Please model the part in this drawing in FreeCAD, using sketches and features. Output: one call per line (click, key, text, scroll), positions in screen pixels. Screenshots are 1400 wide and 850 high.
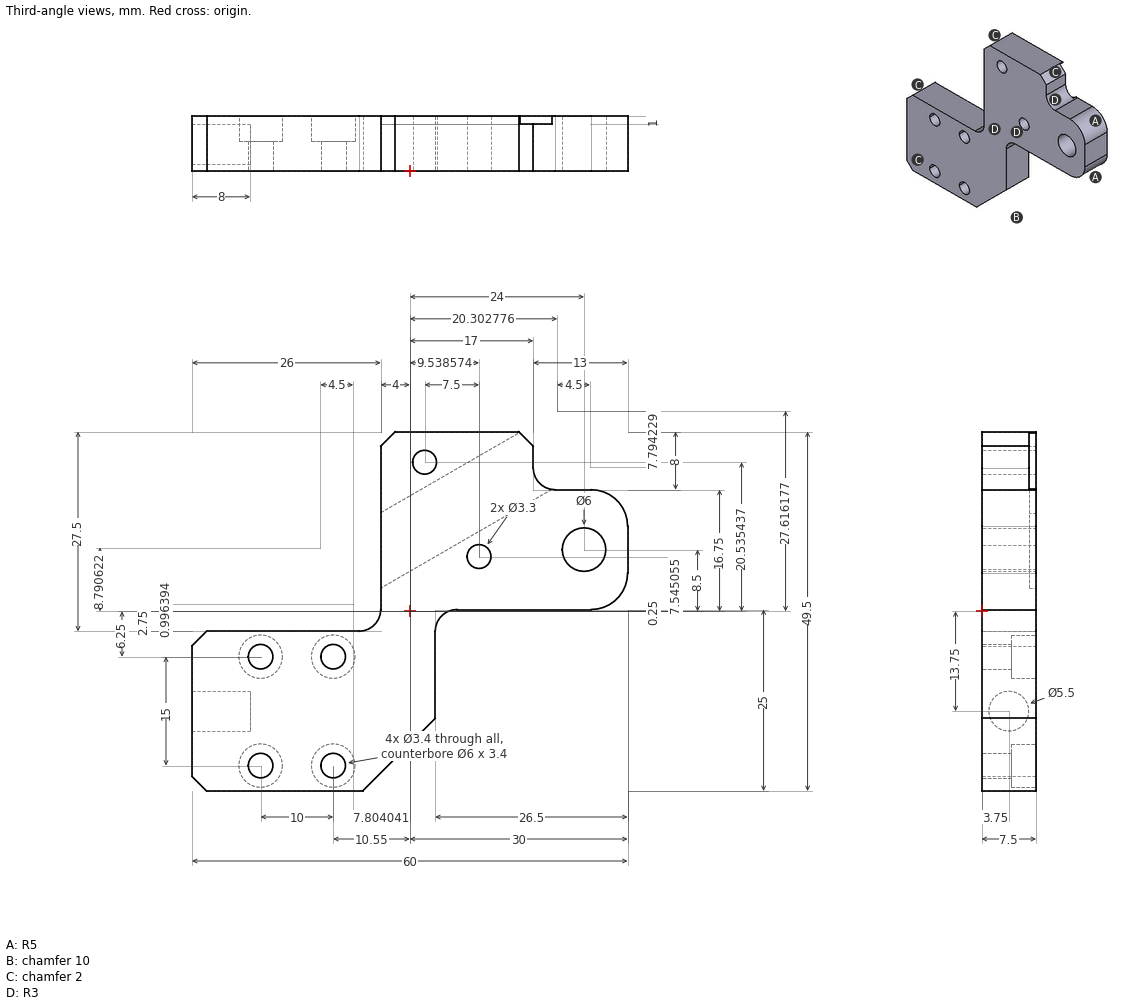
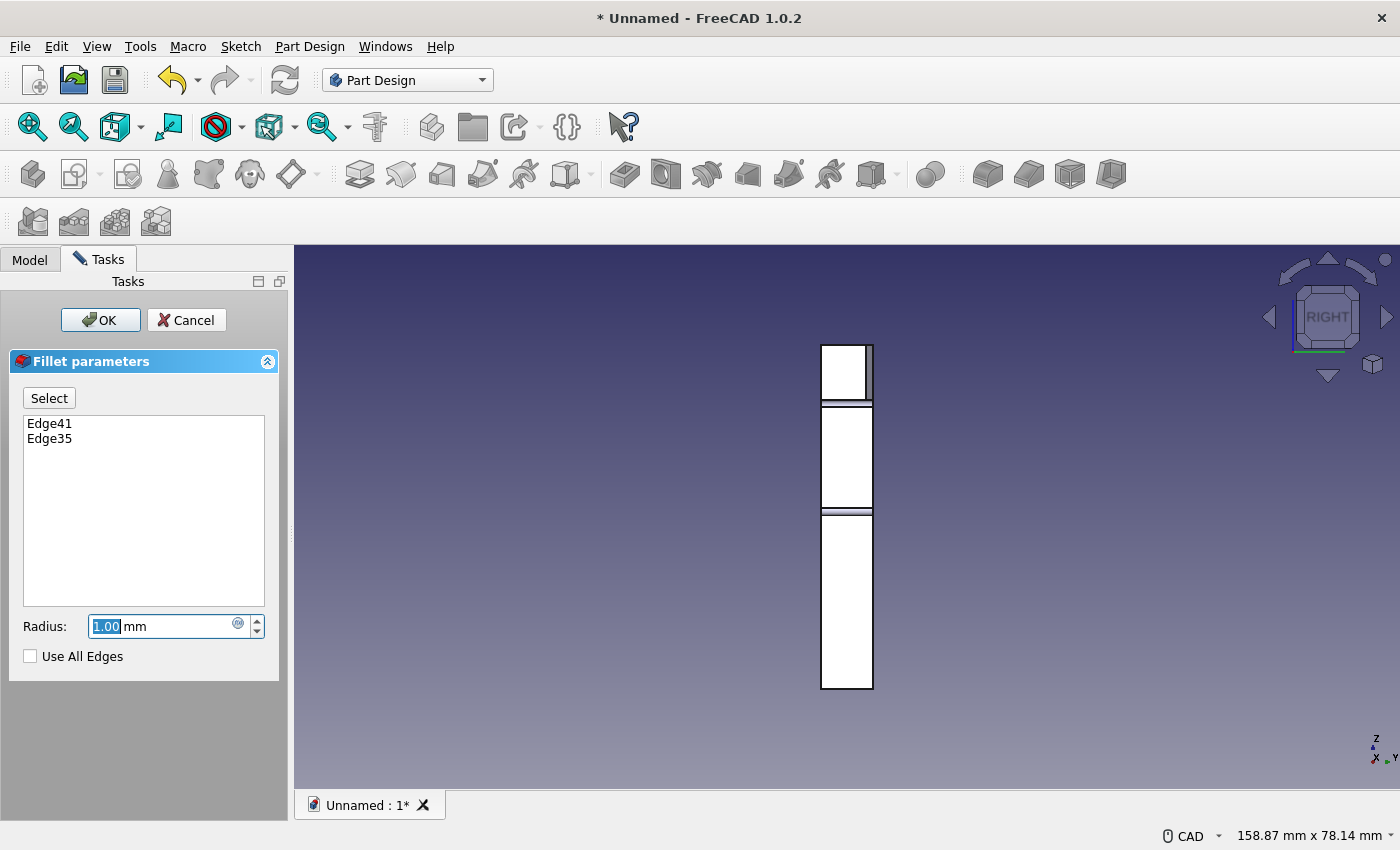
text(5)
key(Tab)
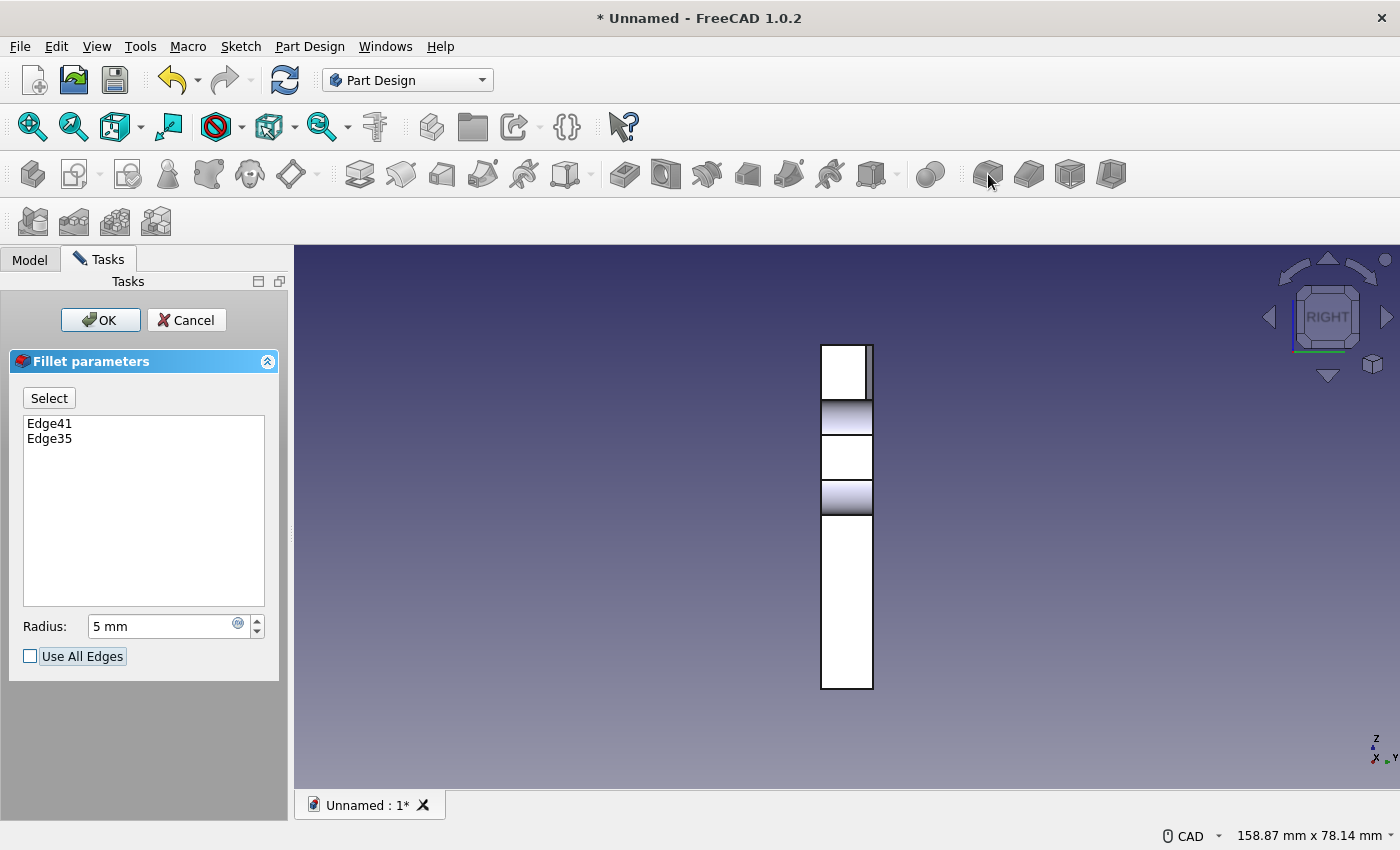
click(101, 320)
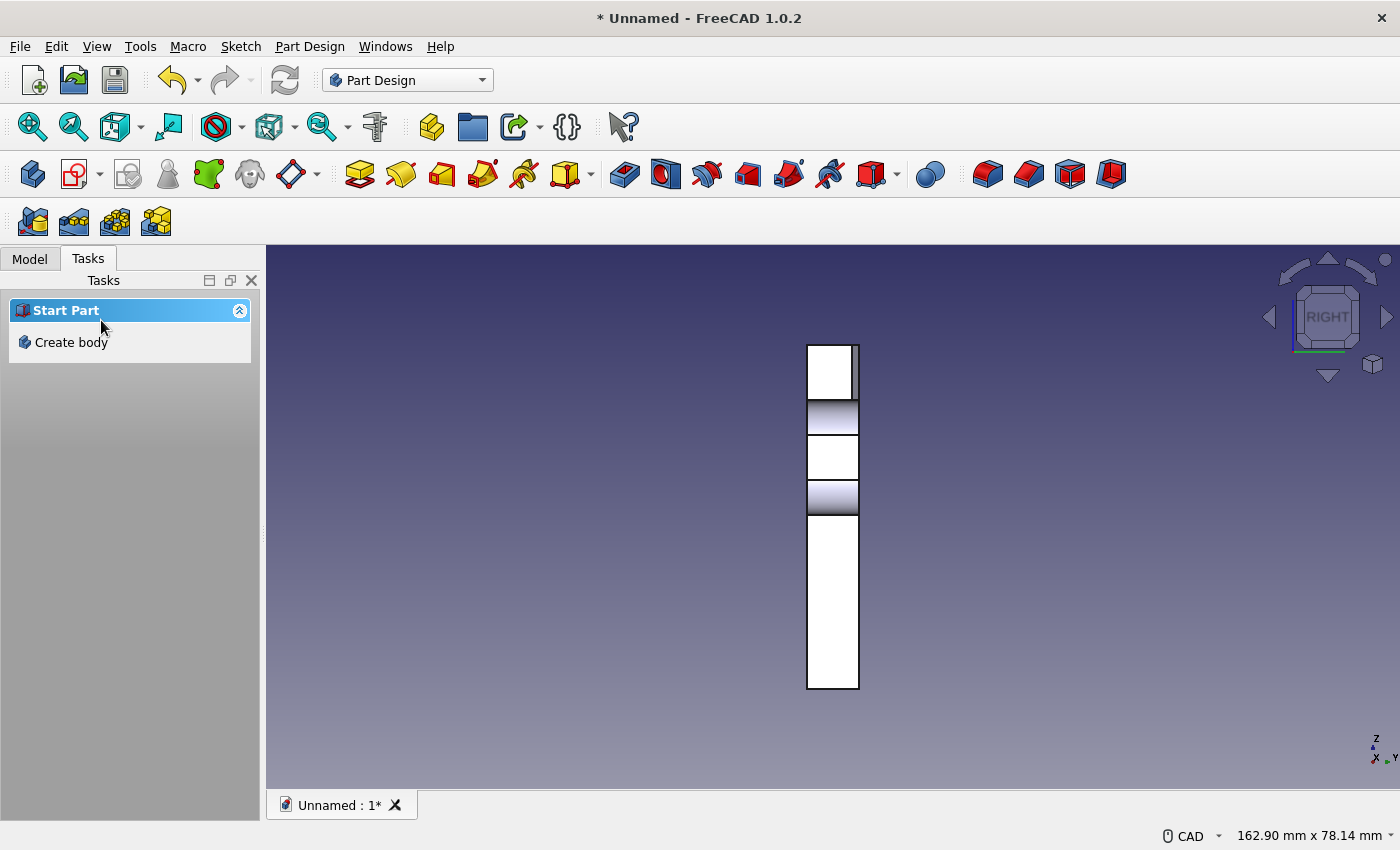
click(833, 688)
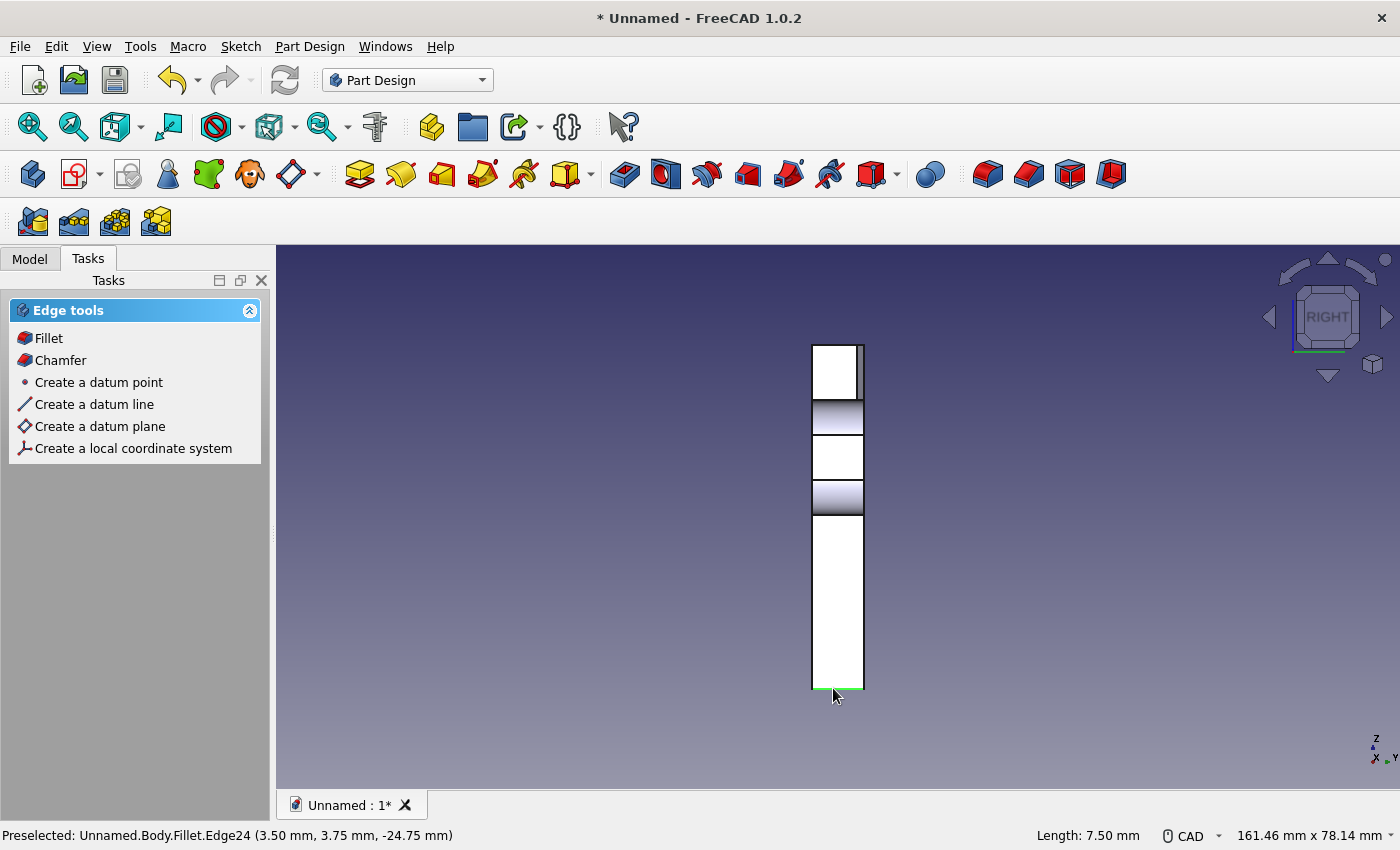
click(1029, 174)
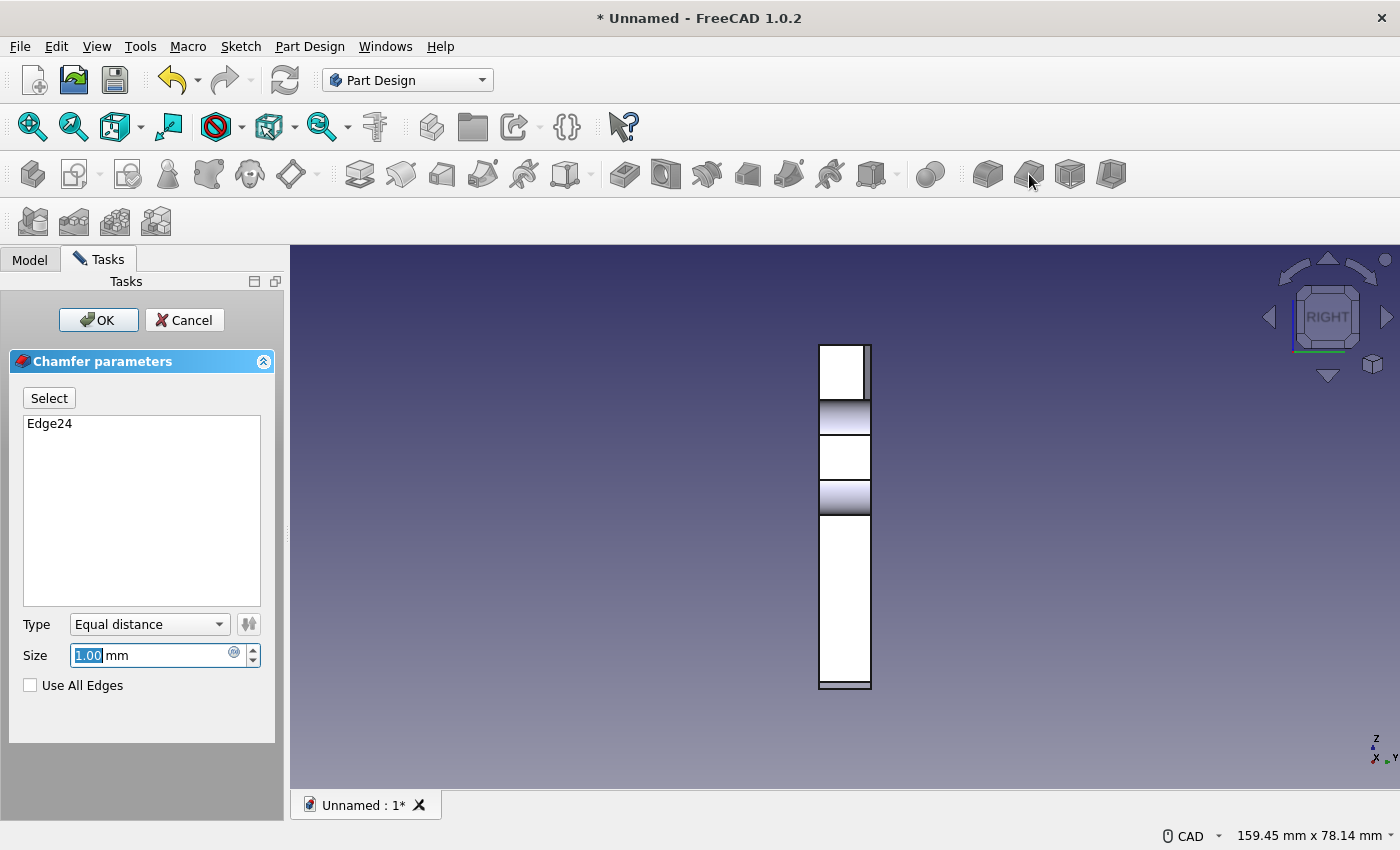
text(10)
key(Tab)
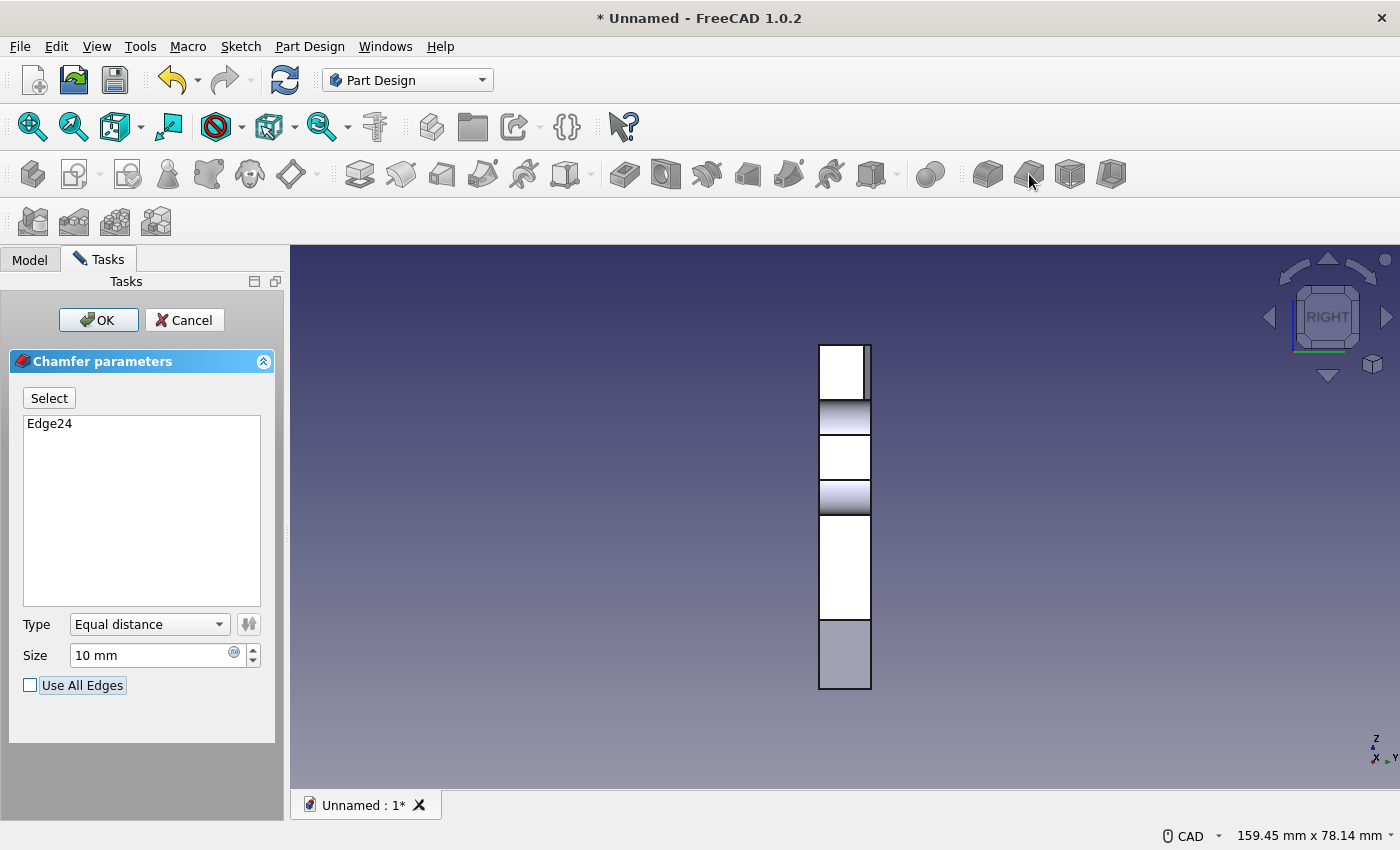
click(99, 320)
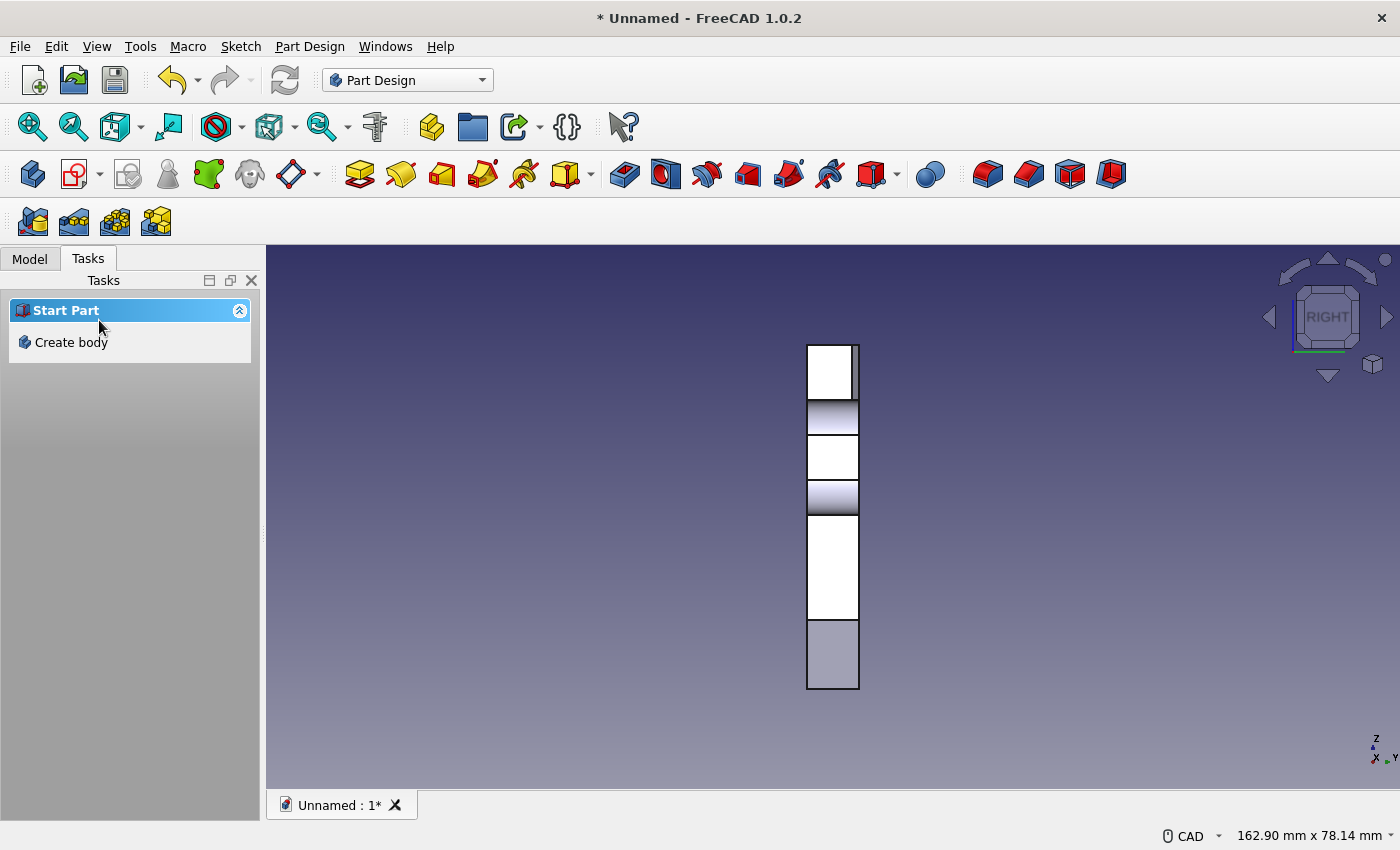
click(830, 344)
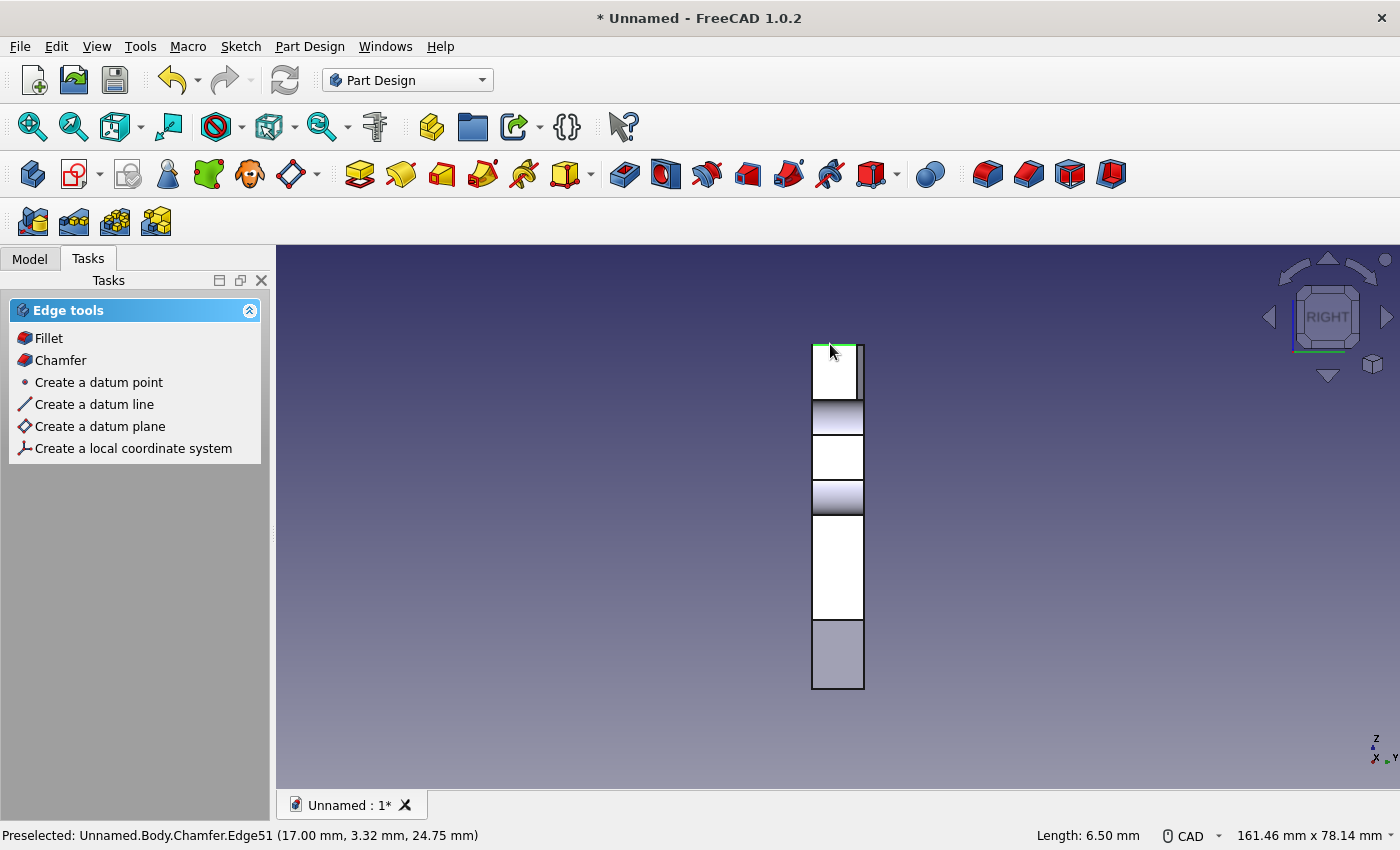
key(0)